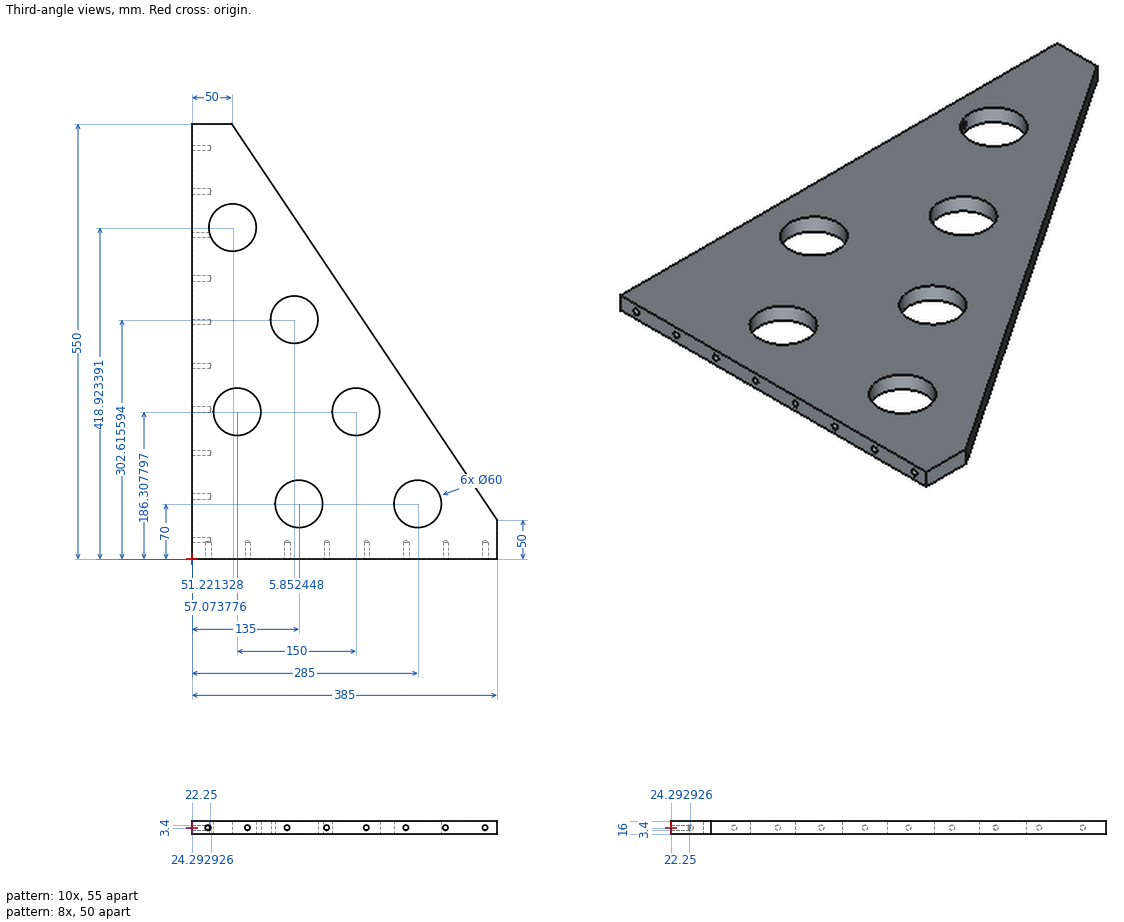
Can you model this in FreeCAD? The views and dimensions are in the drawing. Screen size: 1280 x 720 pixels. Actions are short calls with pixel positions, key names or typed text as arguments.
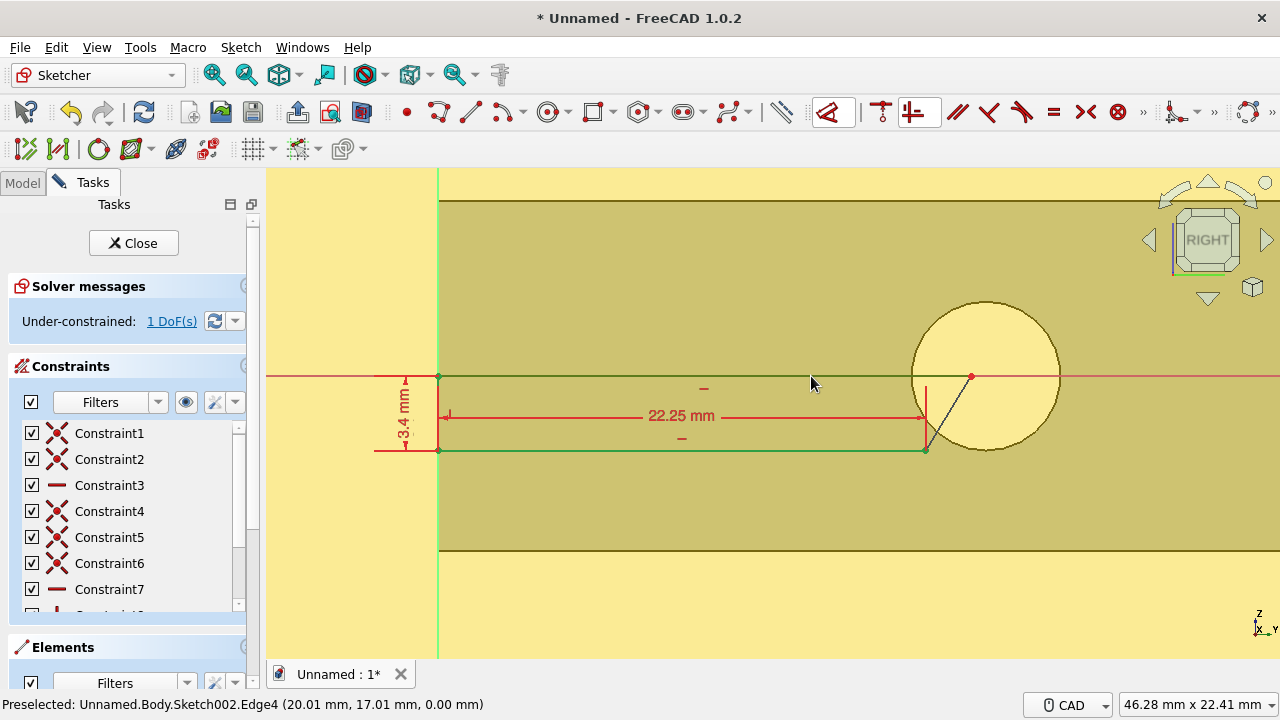
click(850, 112)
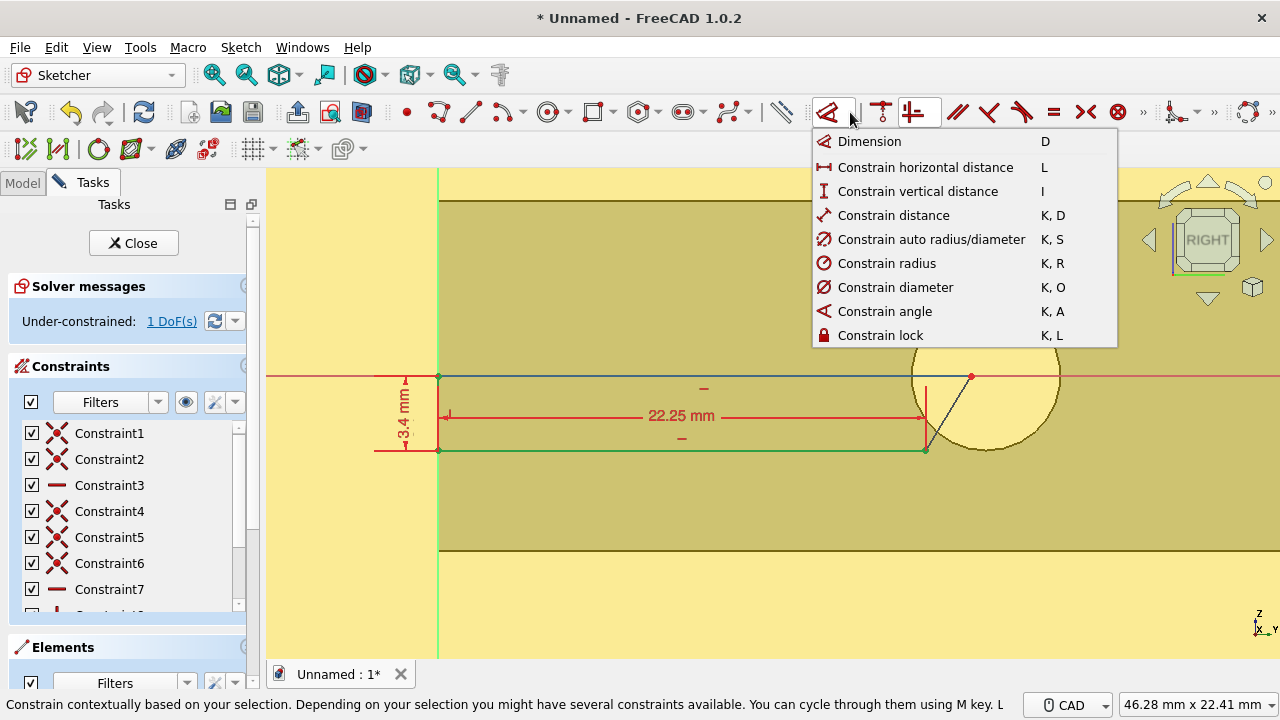
click(965, 167)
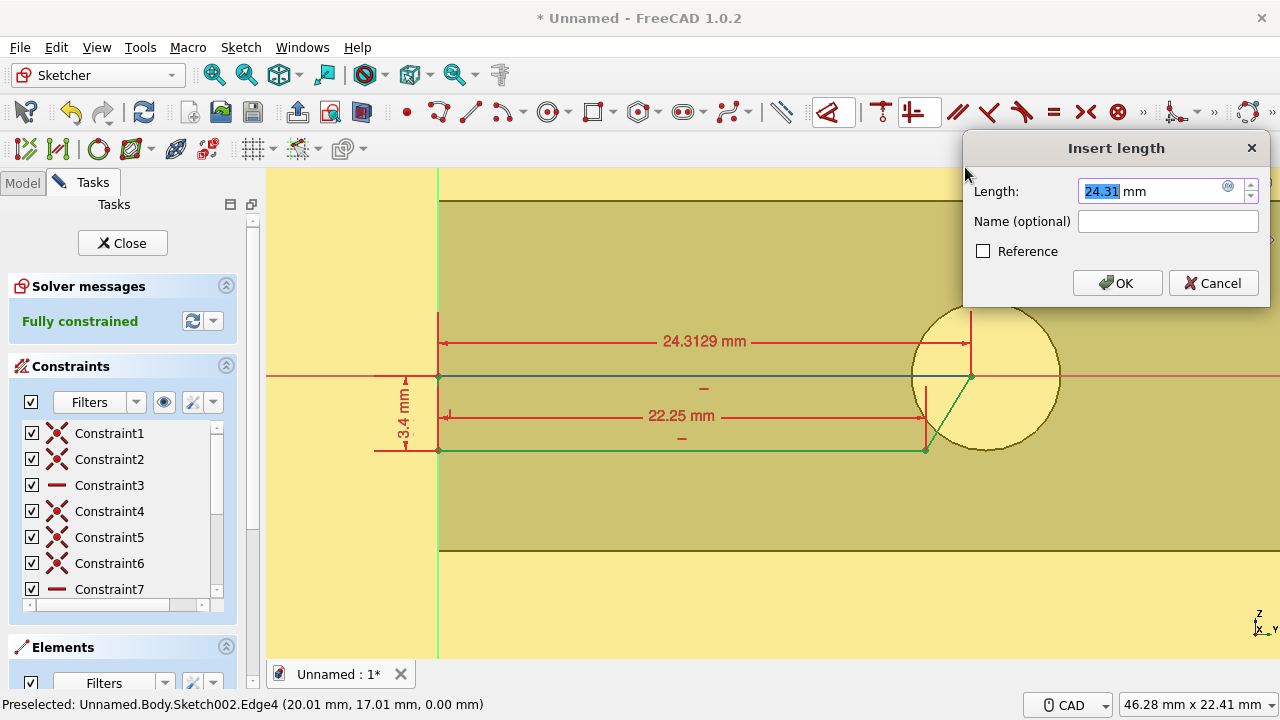
text(24.292926)
key(Return)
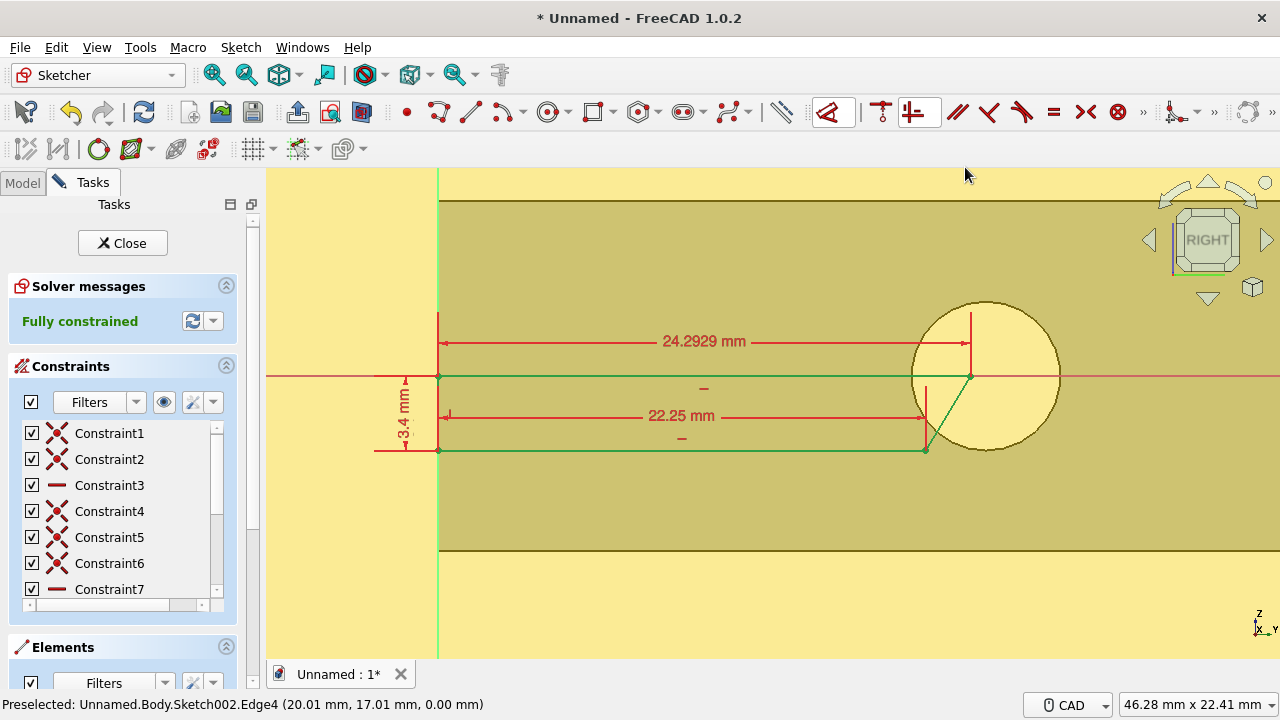
click(123, 243)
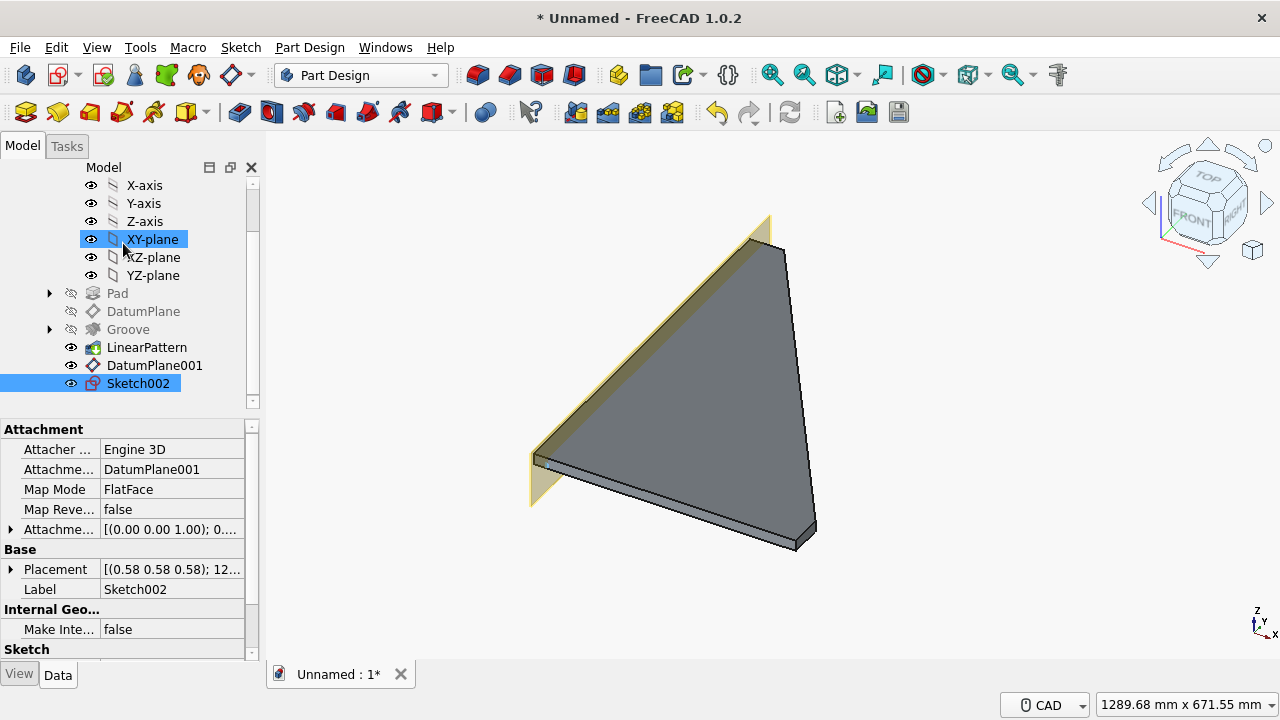
click(304, 112)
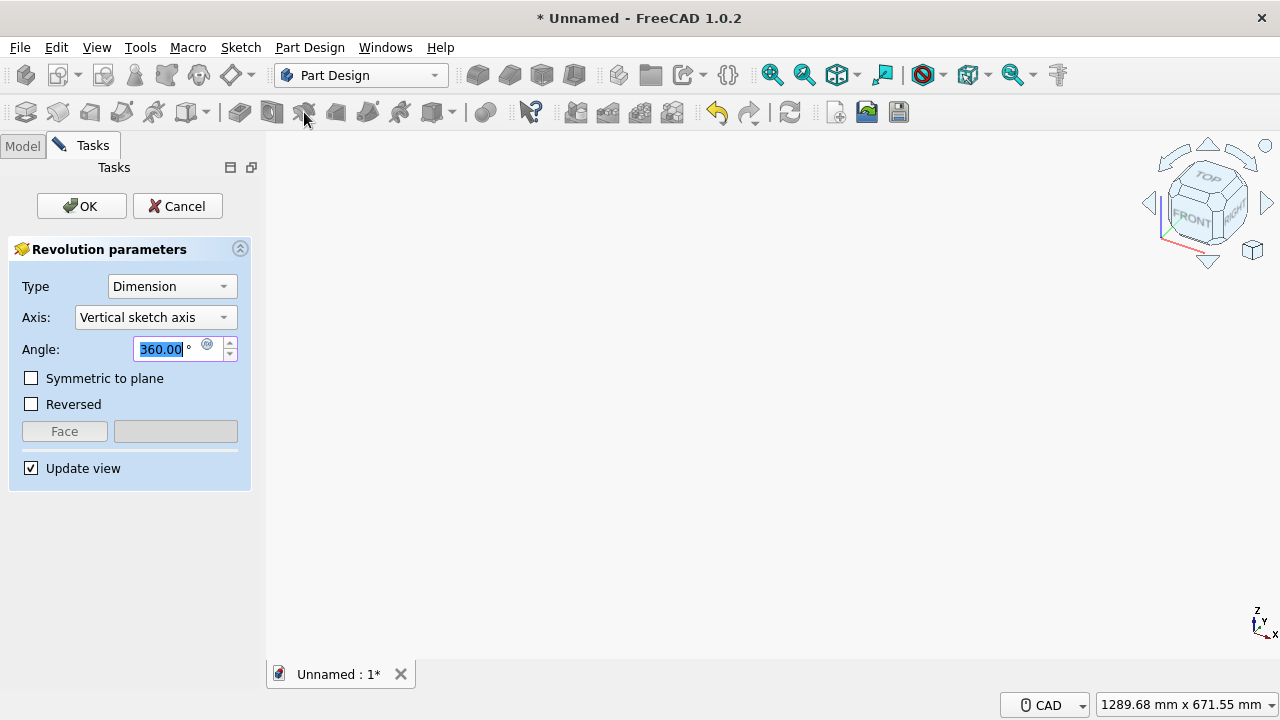
click(156, 318)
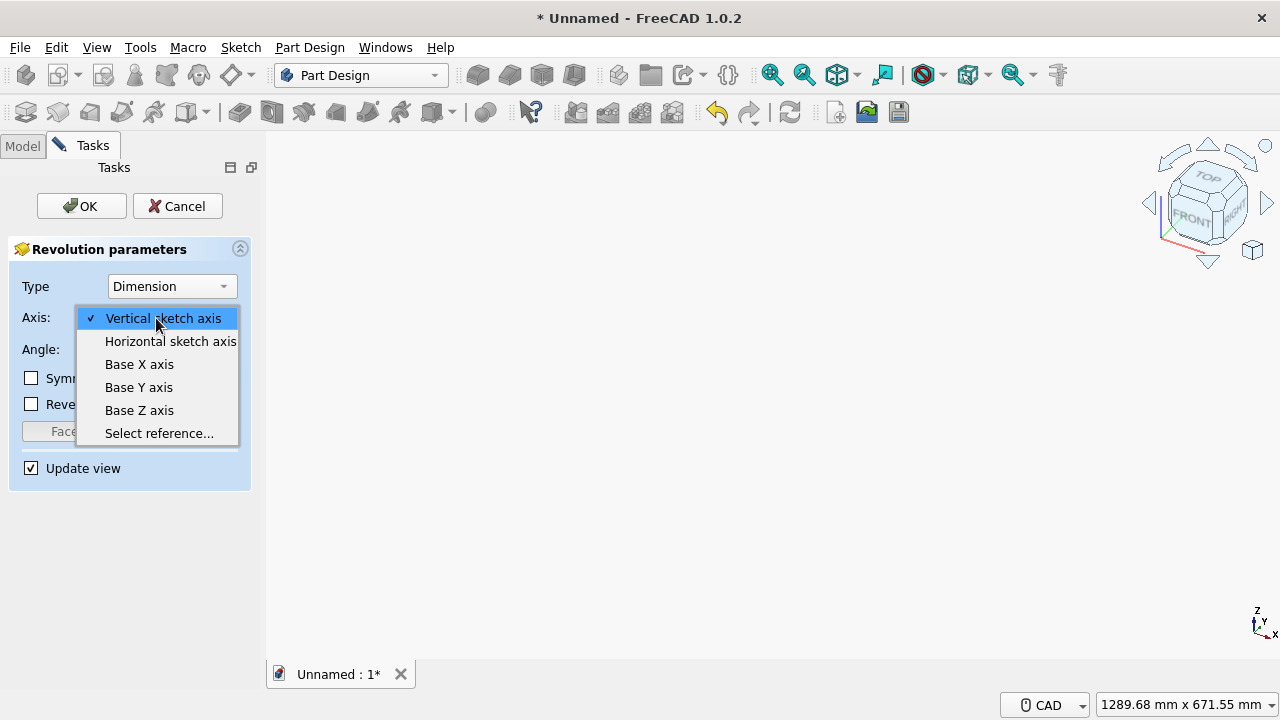
click(156, 342)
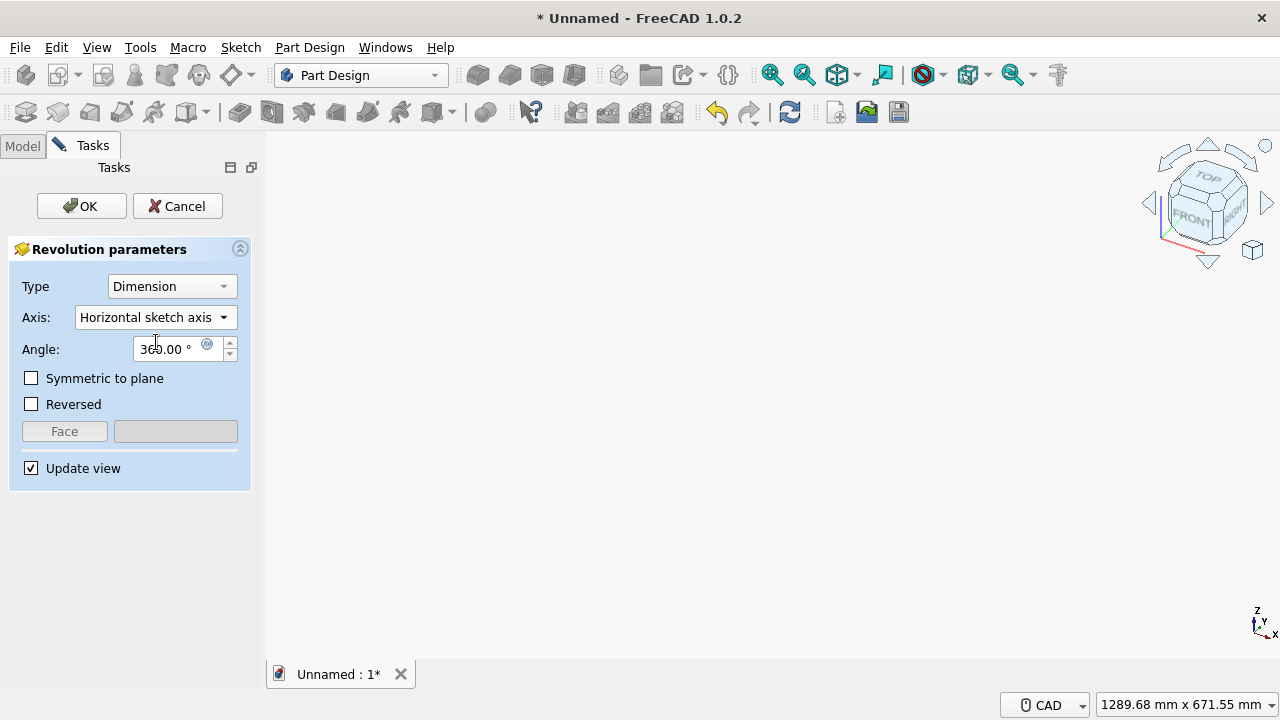
click(82, 206)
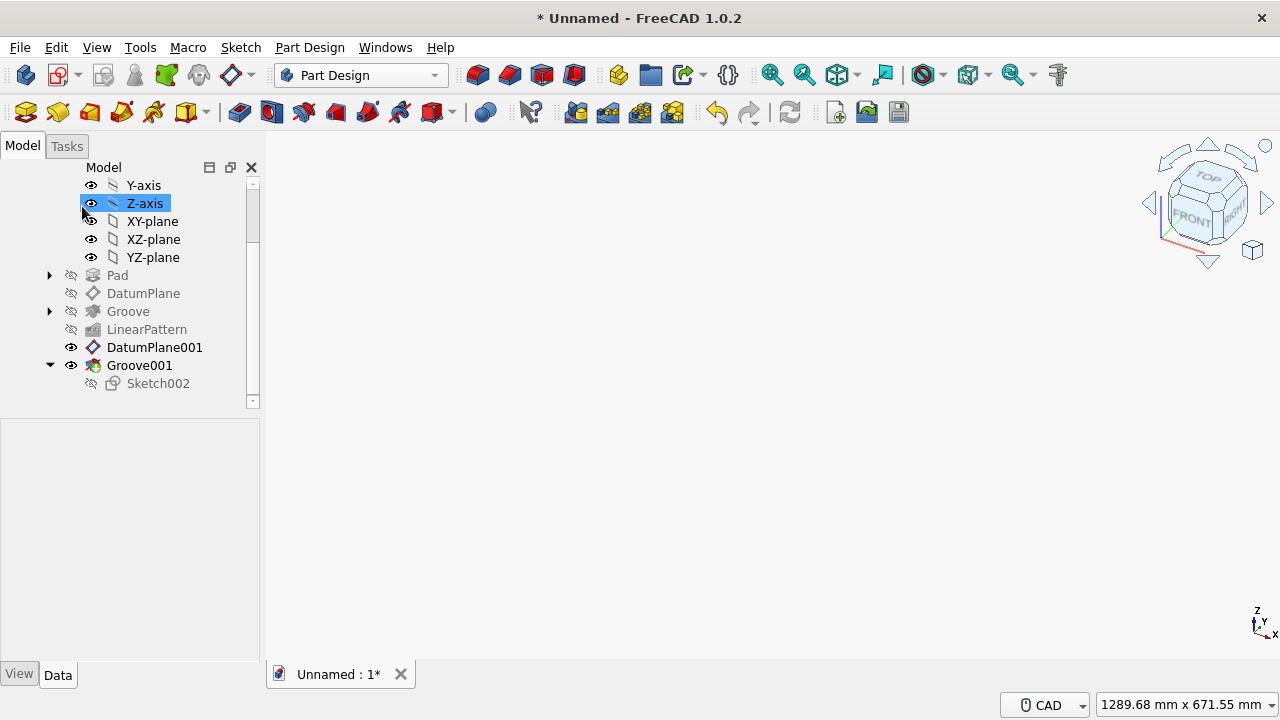
click(116, 347)
key(space)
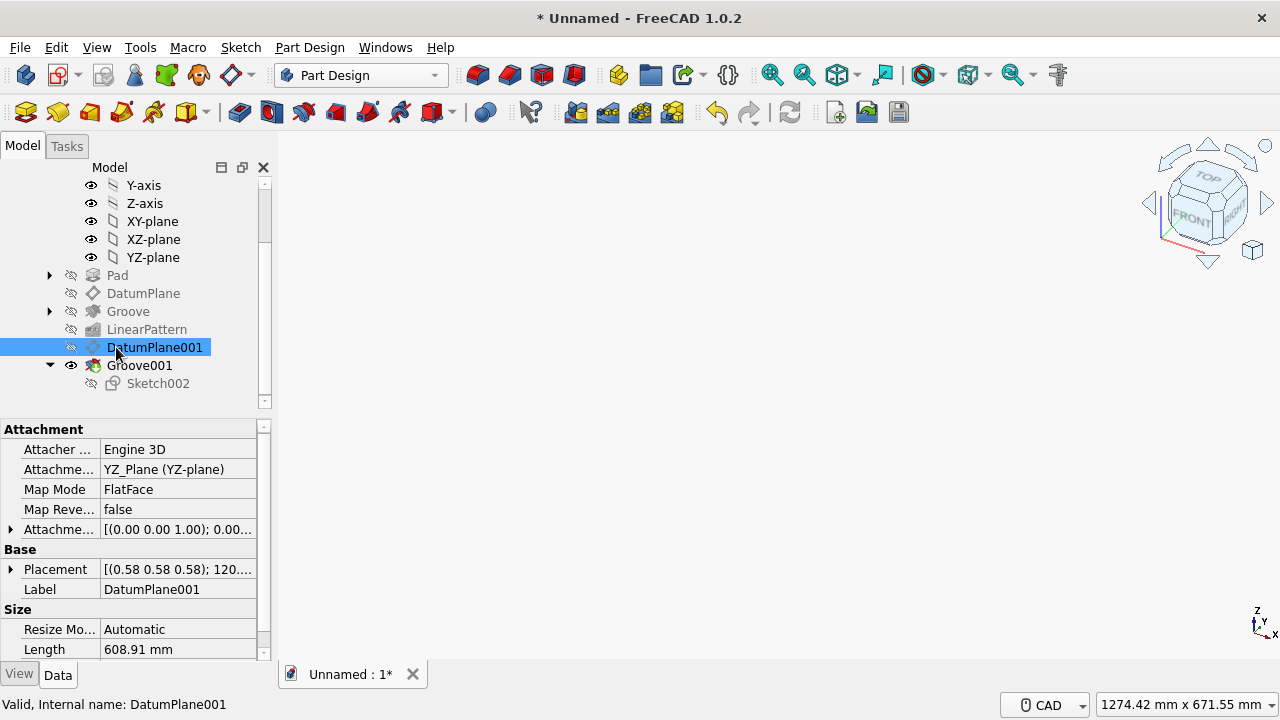
click(774, 76)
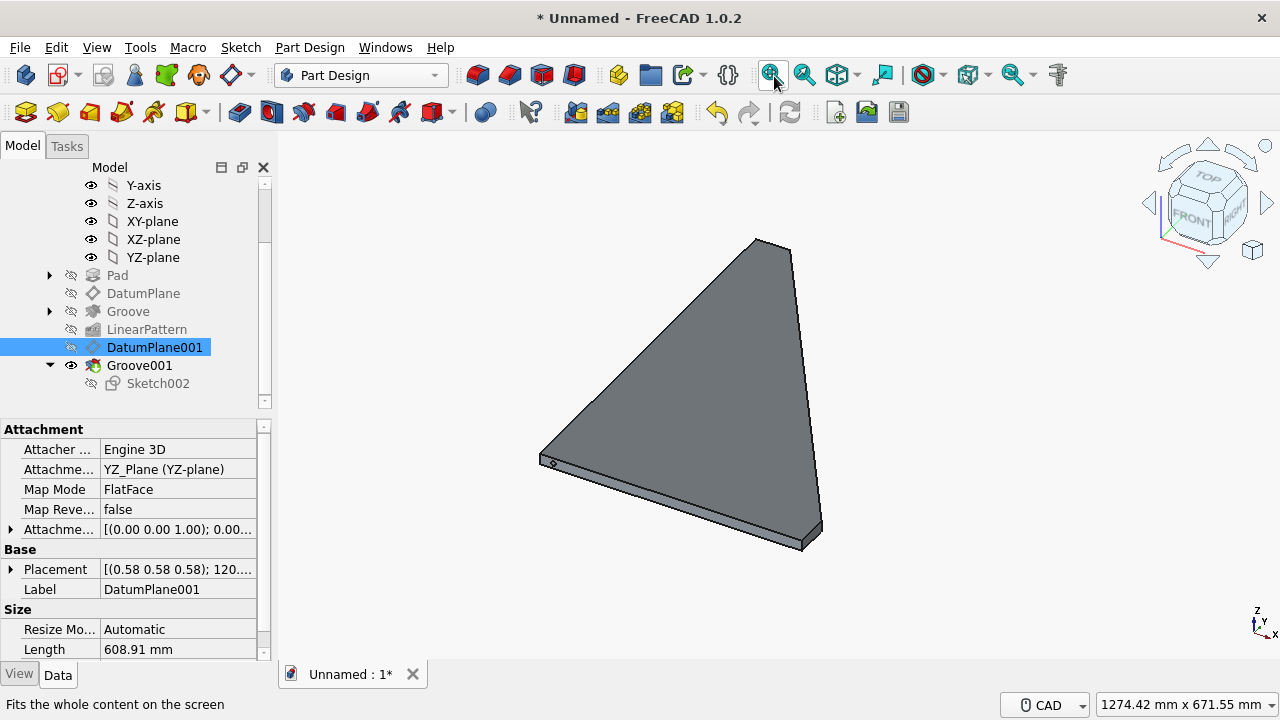
click(116, 365)